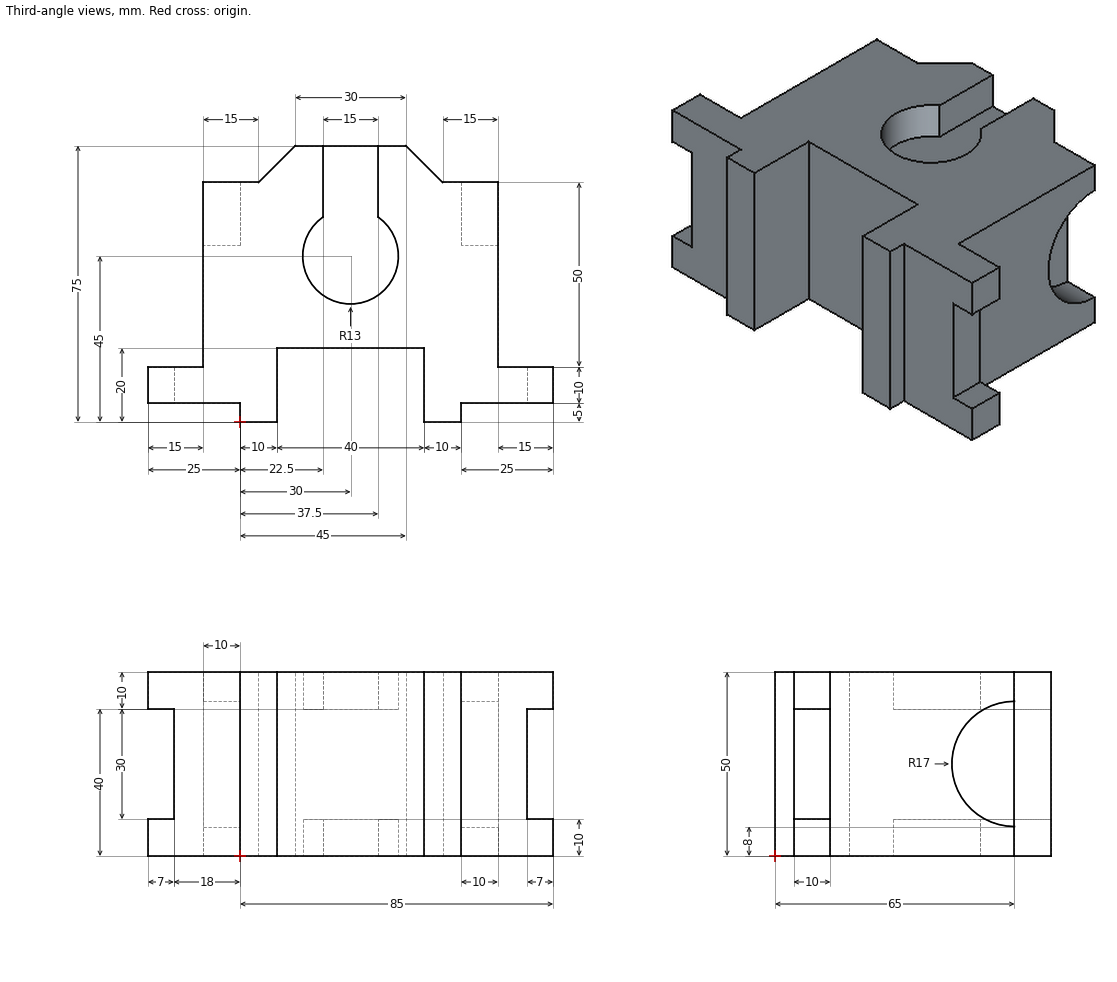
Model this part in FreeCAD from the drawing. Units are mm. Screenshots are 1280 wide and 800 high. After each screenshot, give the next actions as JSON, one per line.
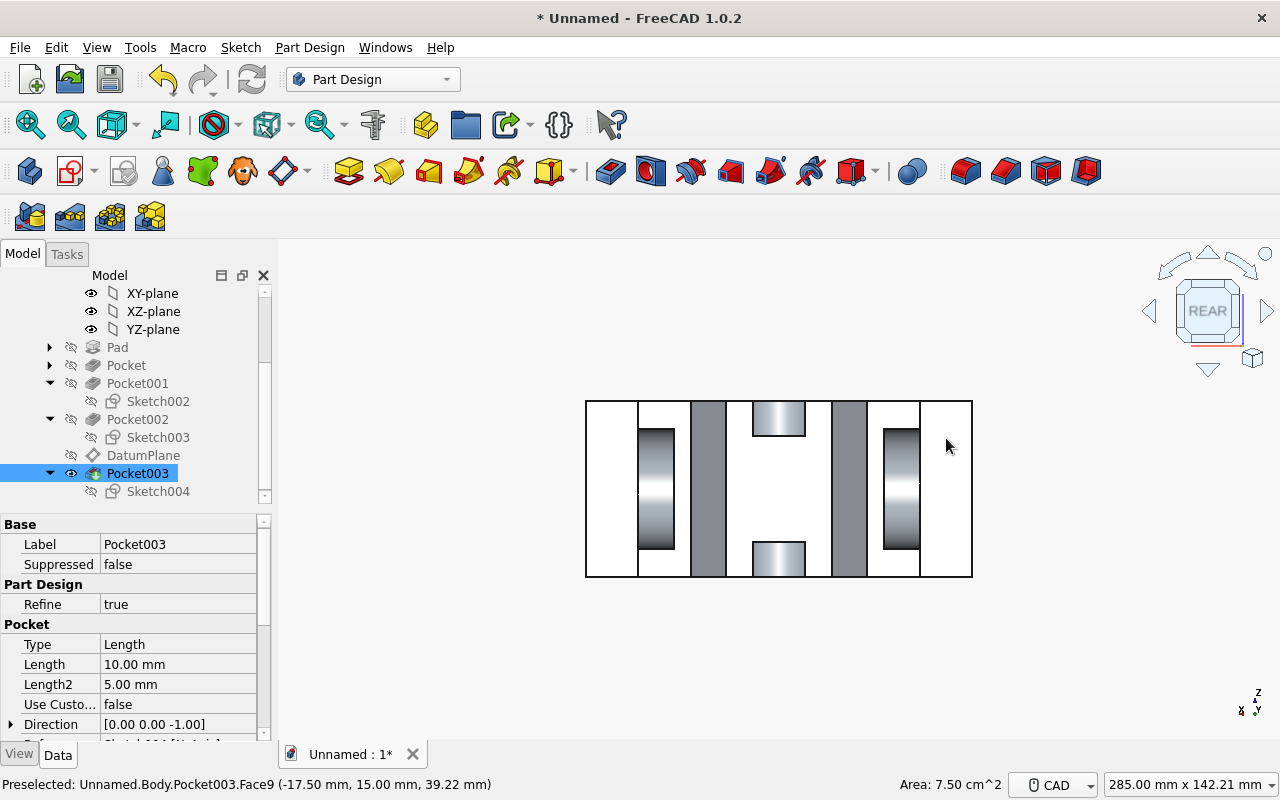
{"action": "left_click", "coordinate": [70, 172]}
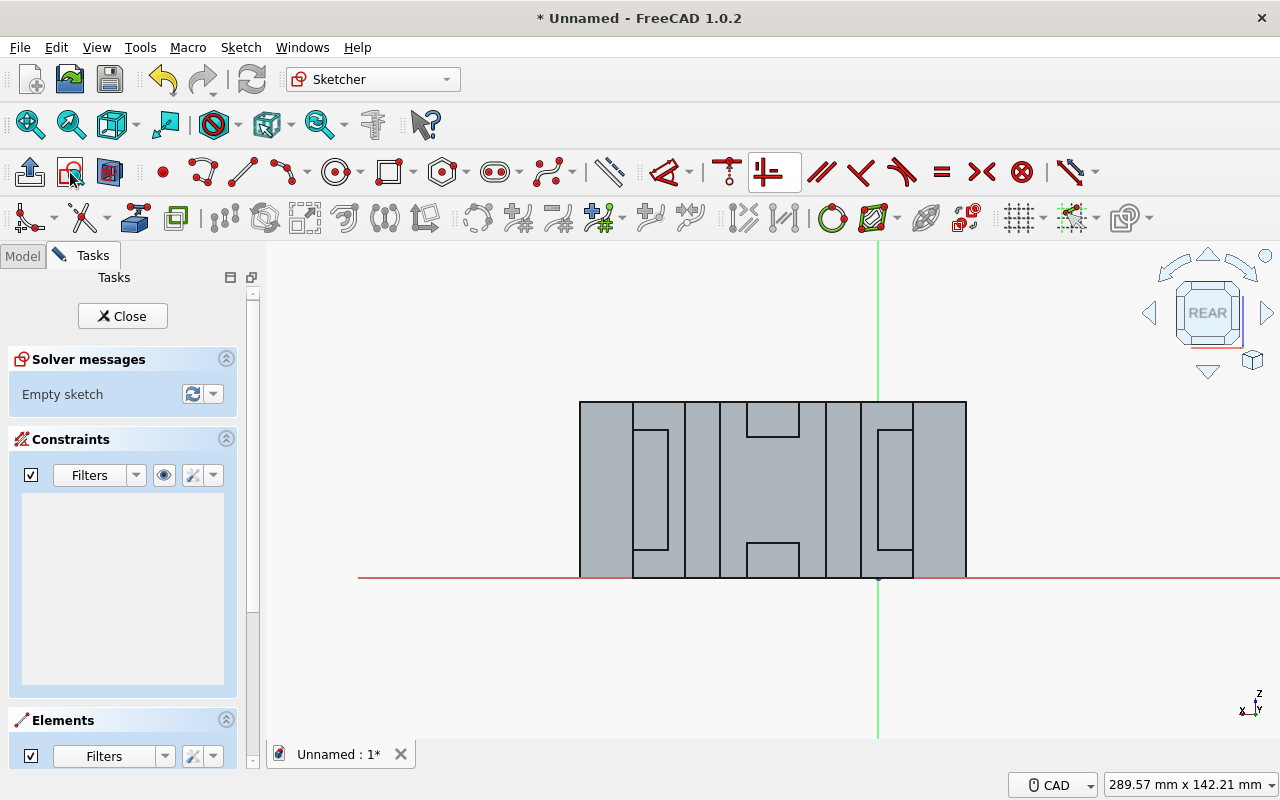
{"action": "scroll", "coordinate": [1099, 522], "scroll_direction": "up", "scroll_amount": 4}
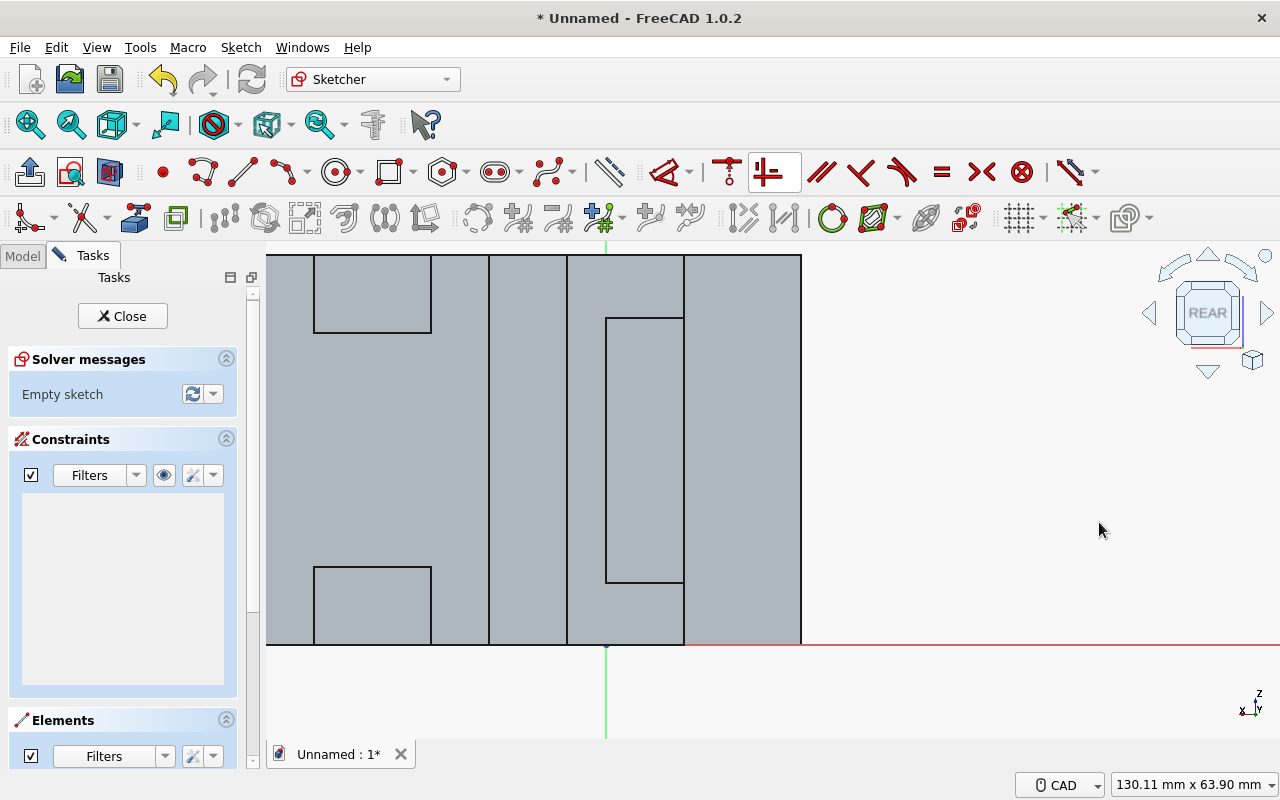
{"action": "left_click", "coordinate": [390, 172]}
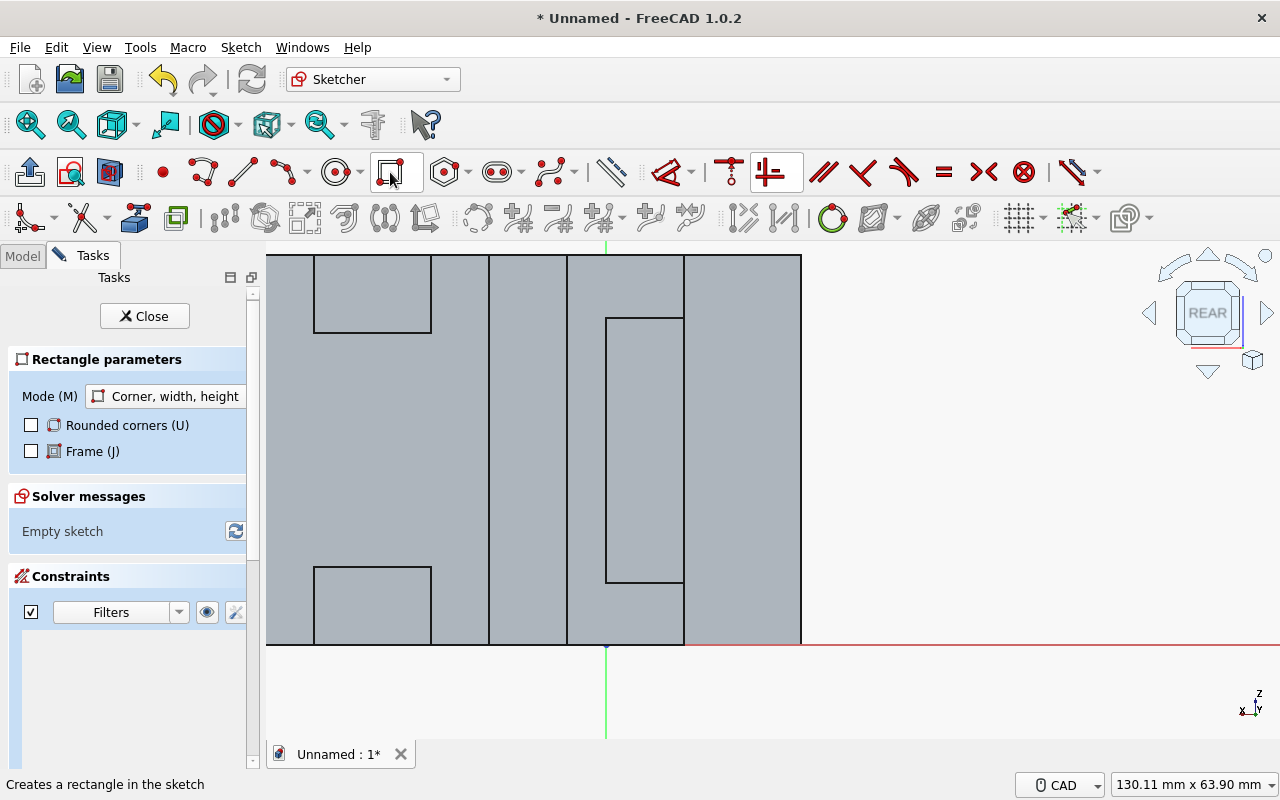
{"action": "left_click", "coordinate": [747, 333]}
{"action": "left_click", "coordinate": [801, 567]}
{"action": "key", "text": "Escape"}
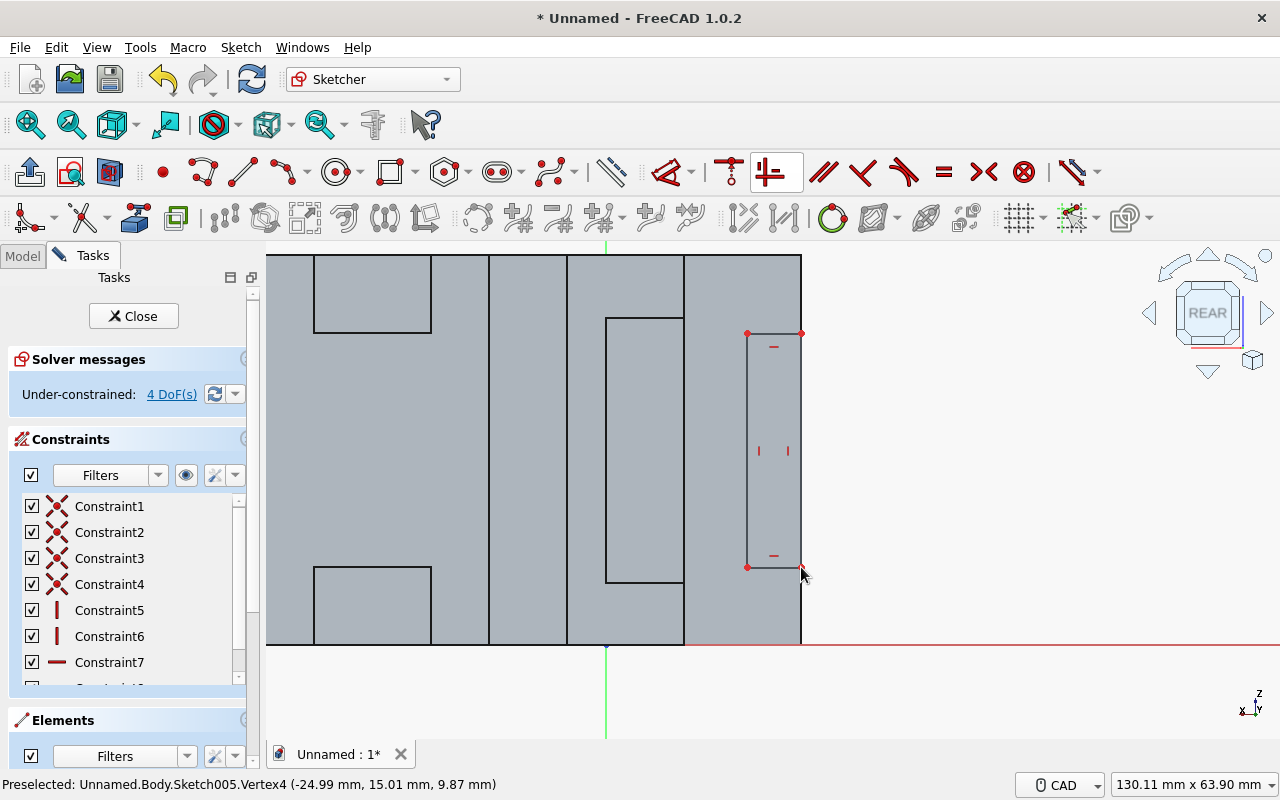
{"action": "left_click", "coordinate": [666, 172]}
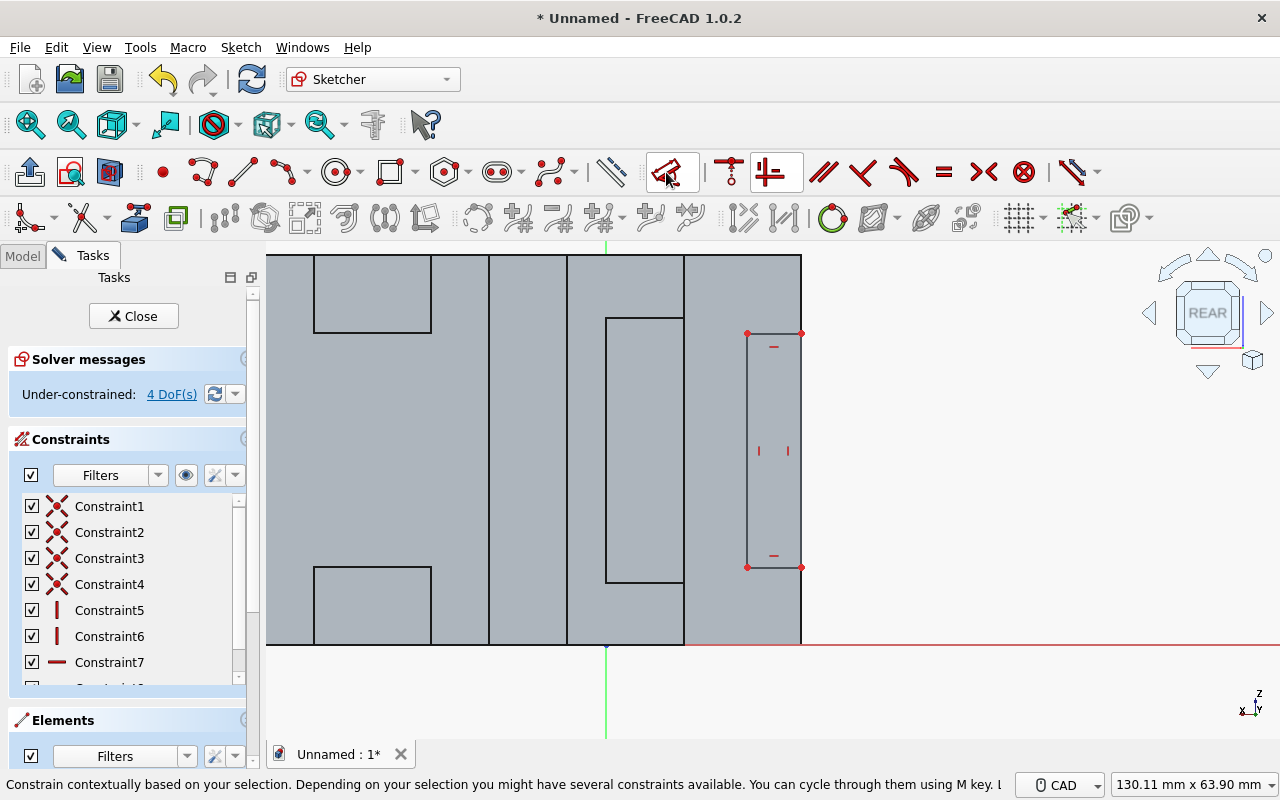
{"action": "left_click", "coordinate": [763, 568]}
{"action": "left_click", "coordinate": [774, 602]}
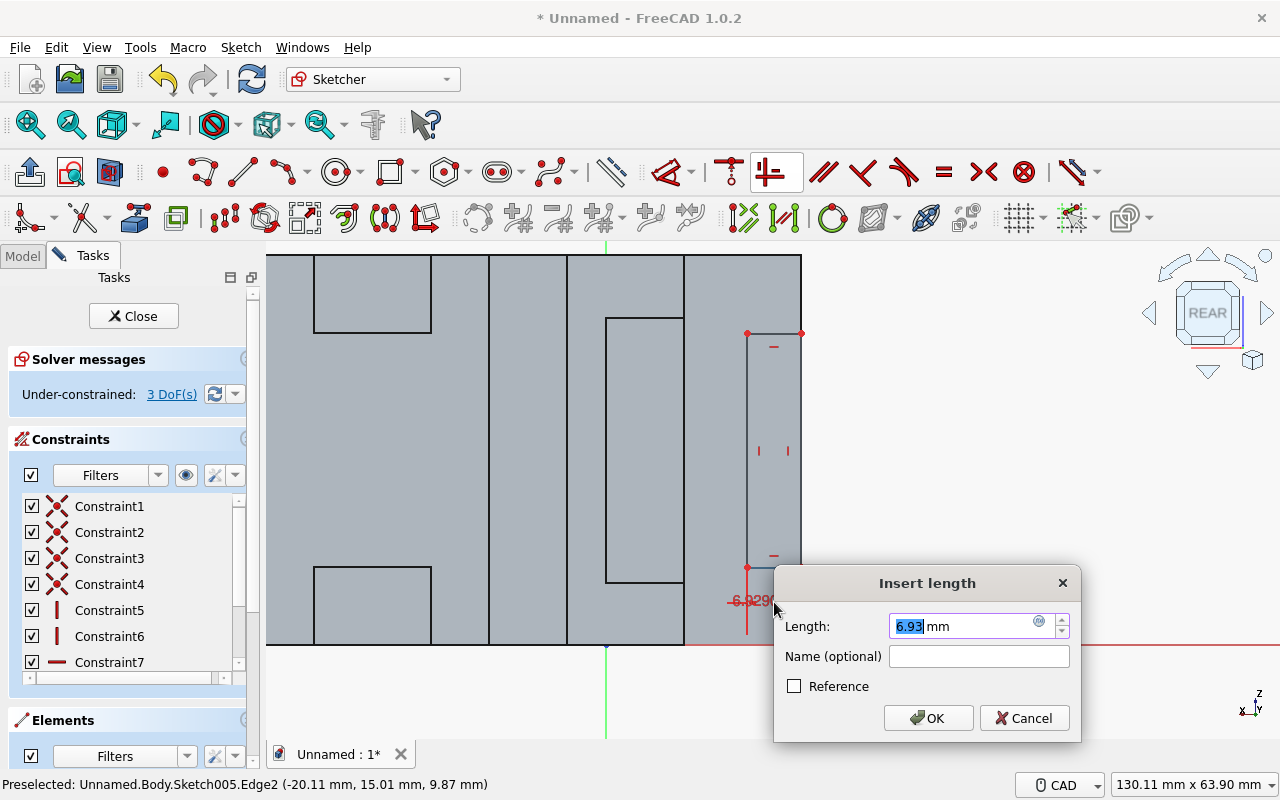
{"action": "type", "text": "7"}
{"action": "key", "text": "Return"}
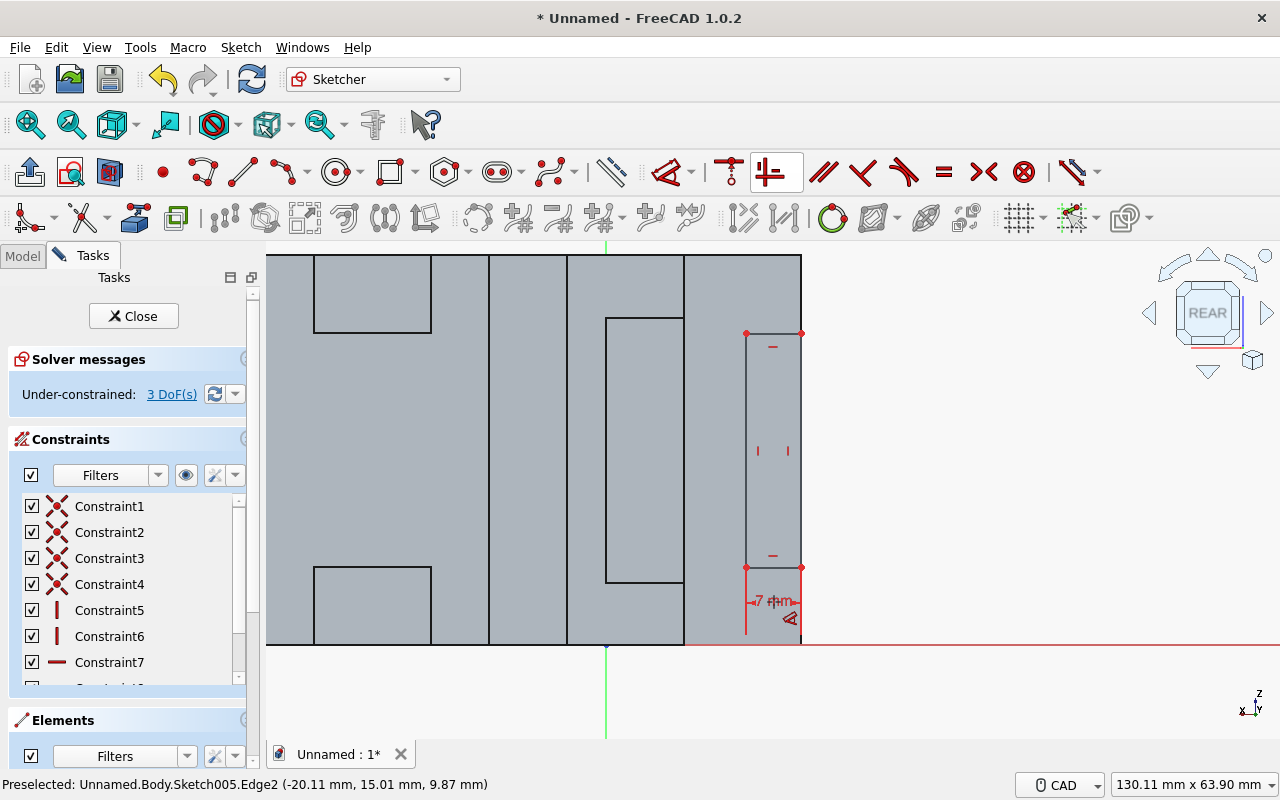
{"action": "left_click", "coordinate": [746, 404]}
{"action": "left_click", "coordinate": [780, 451]}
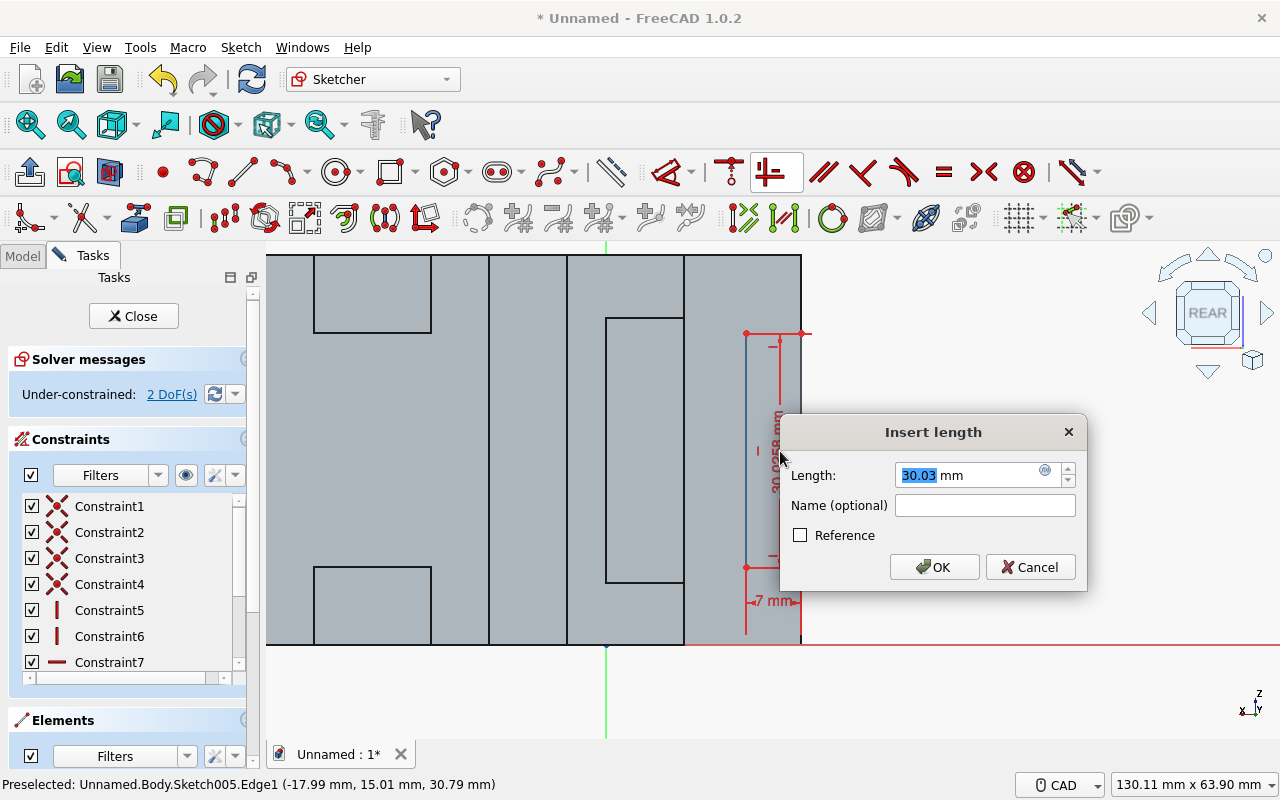
{"action": "type", "text": "30"}
{"action": "key", "text": "Return"}